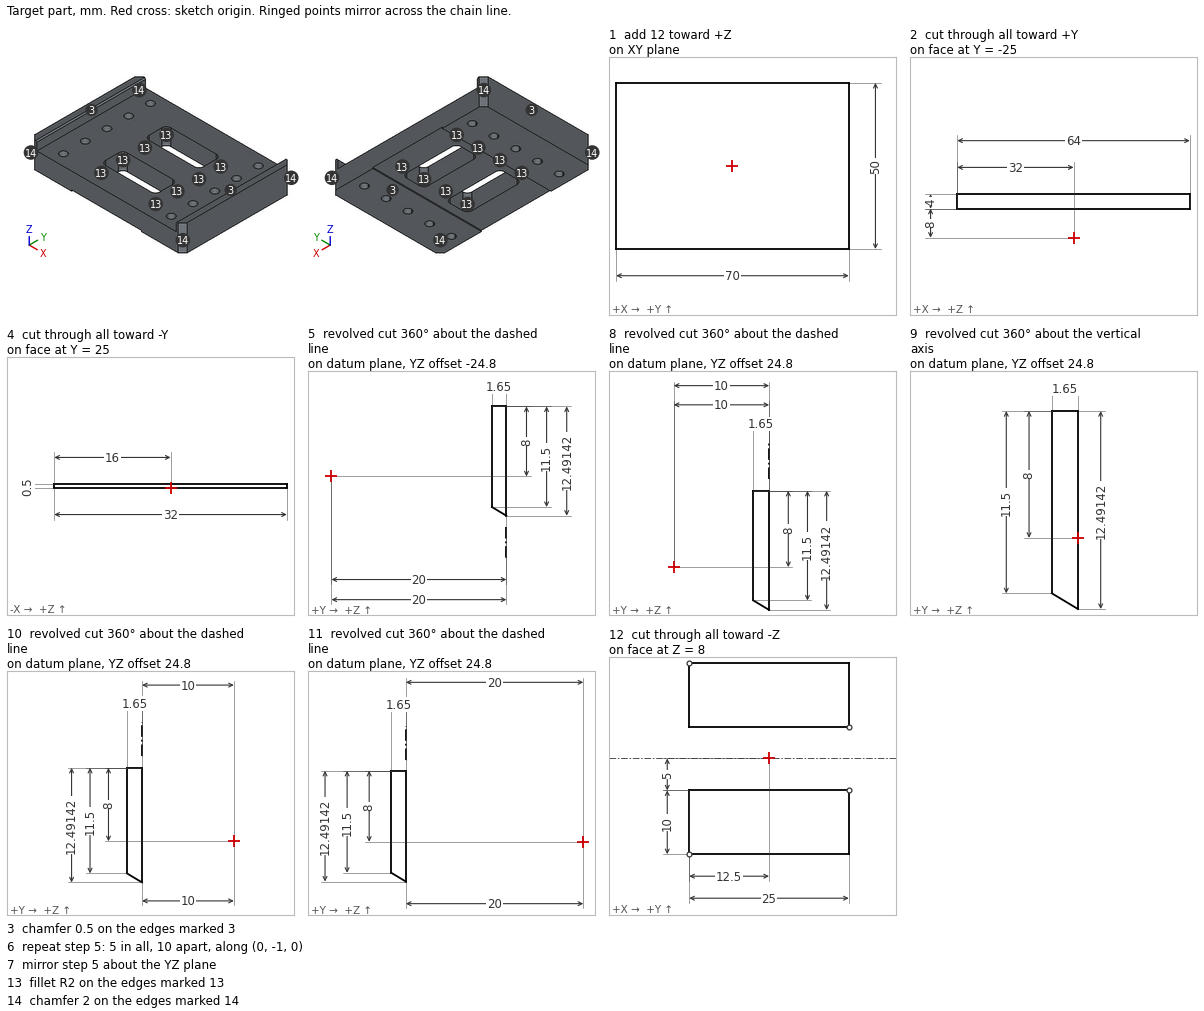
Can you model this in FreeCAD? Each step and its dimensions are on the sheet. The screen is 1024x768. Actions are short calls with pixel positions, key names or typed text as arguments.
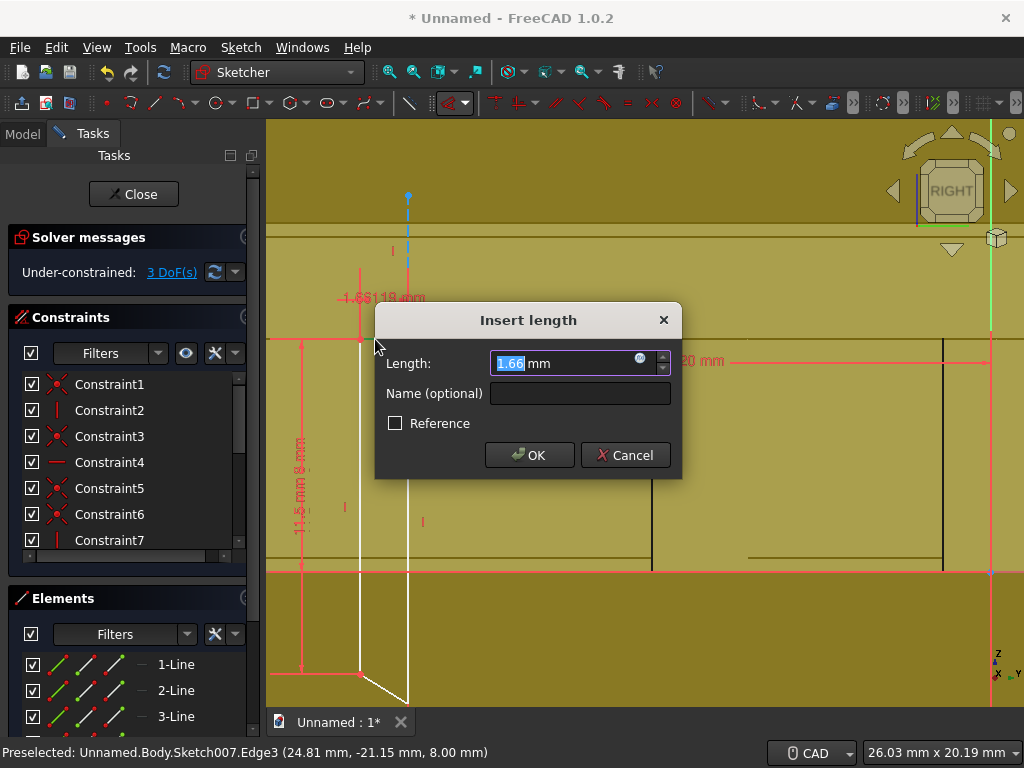
text(1.65)
key(Return)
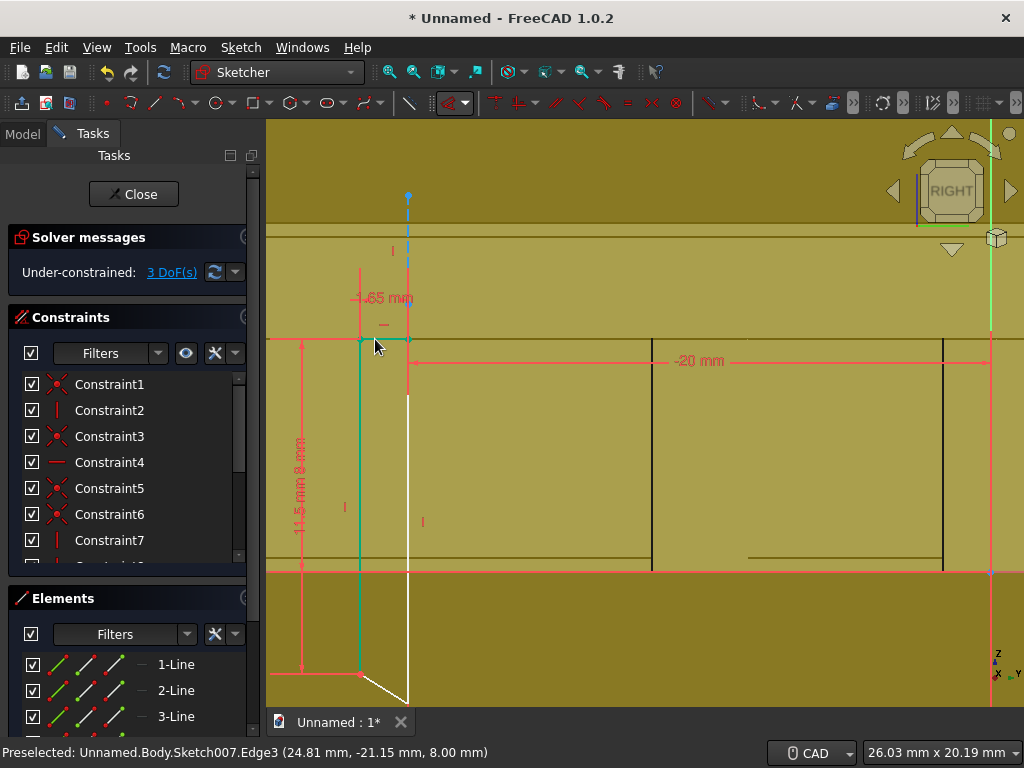
click(408, 449)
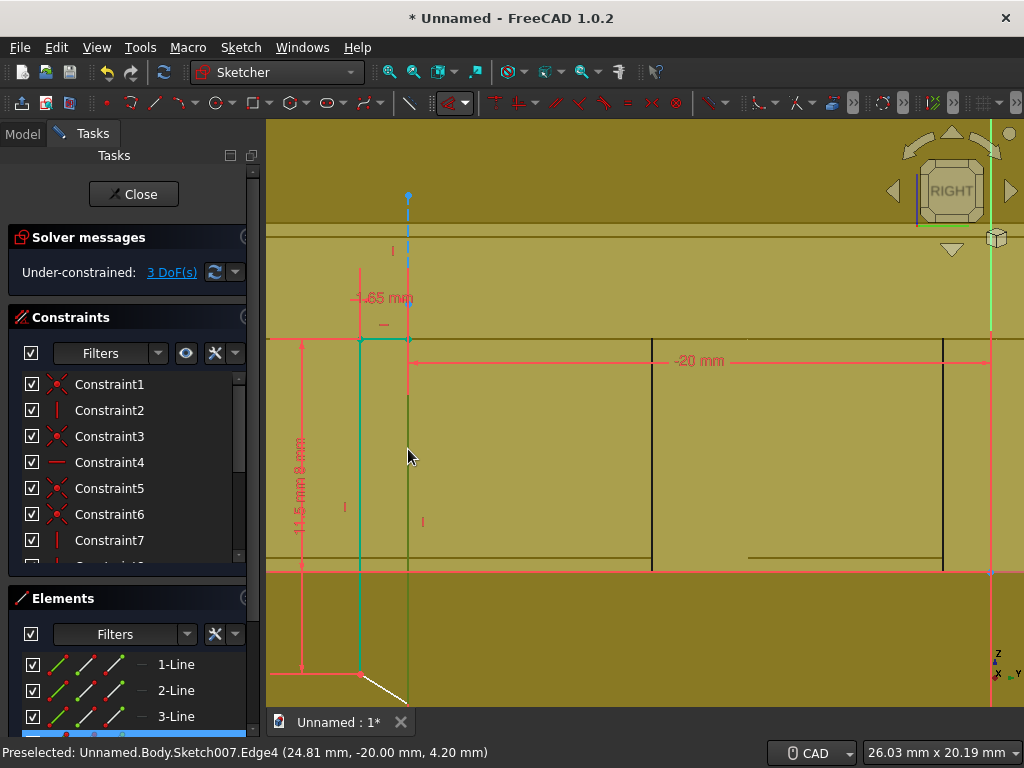
click(468, 104)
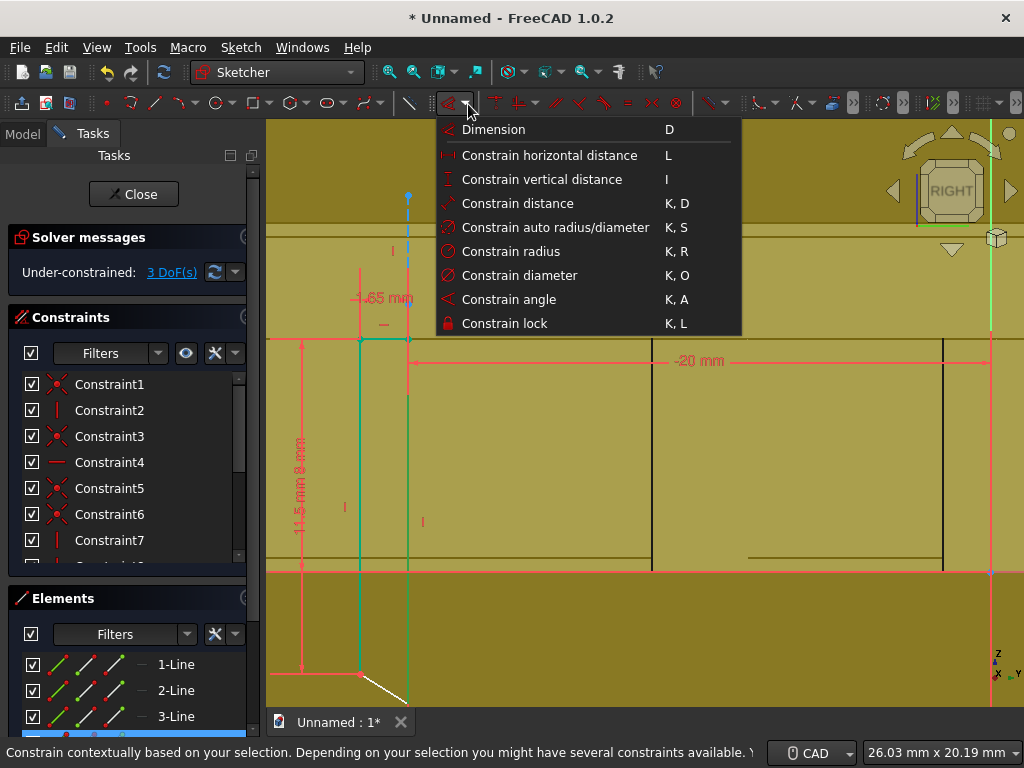
click(589, 179)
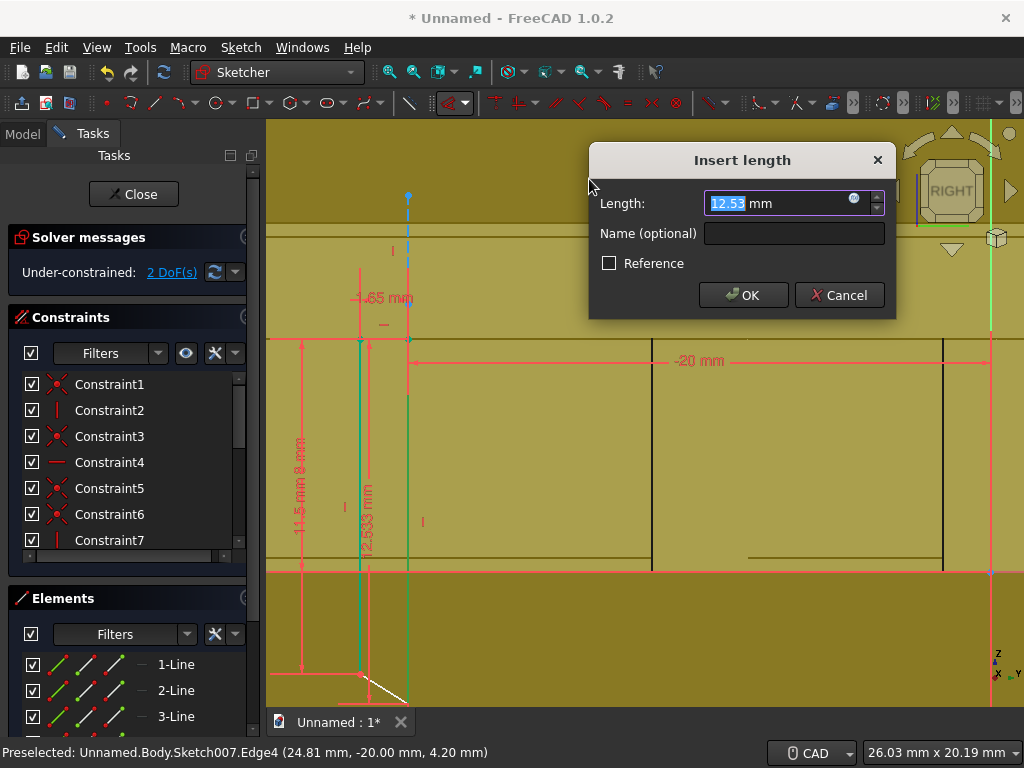
text(12.49142)
key(Return)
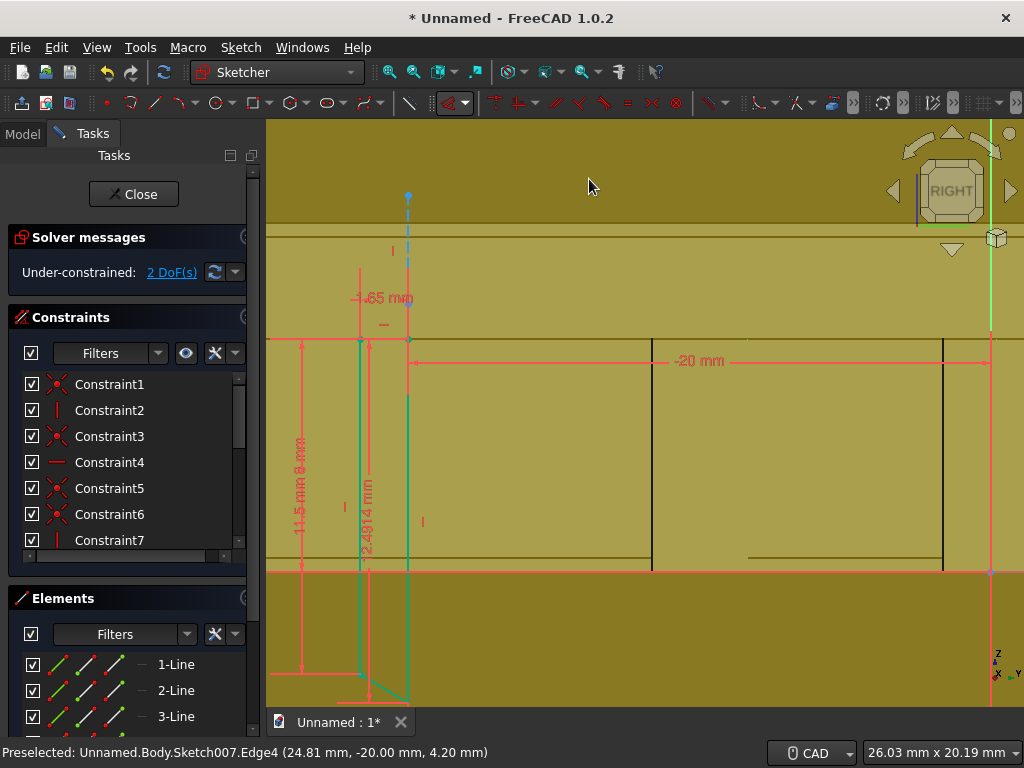
click(134, 194)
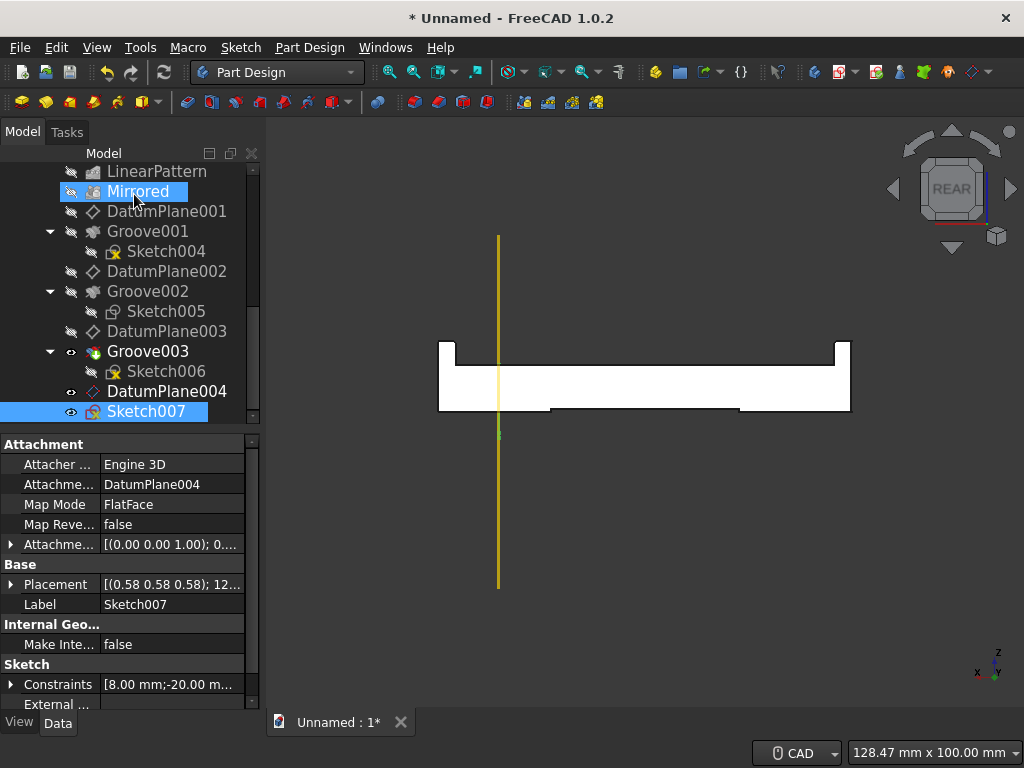
click(236, 102)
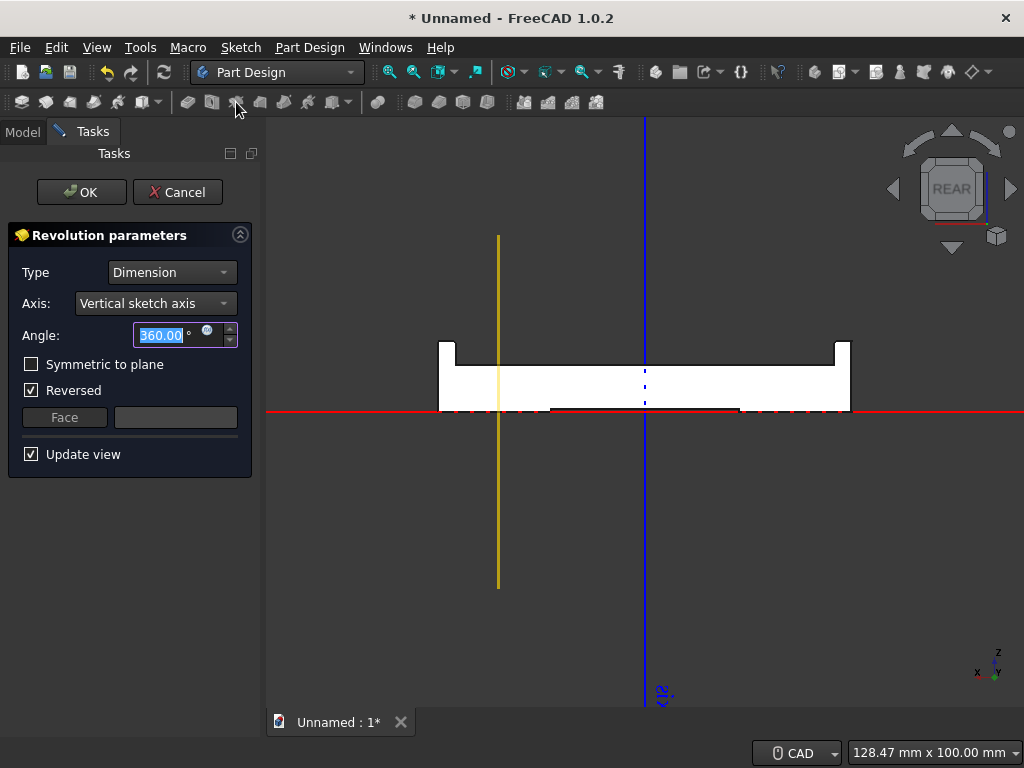
click(156, 304)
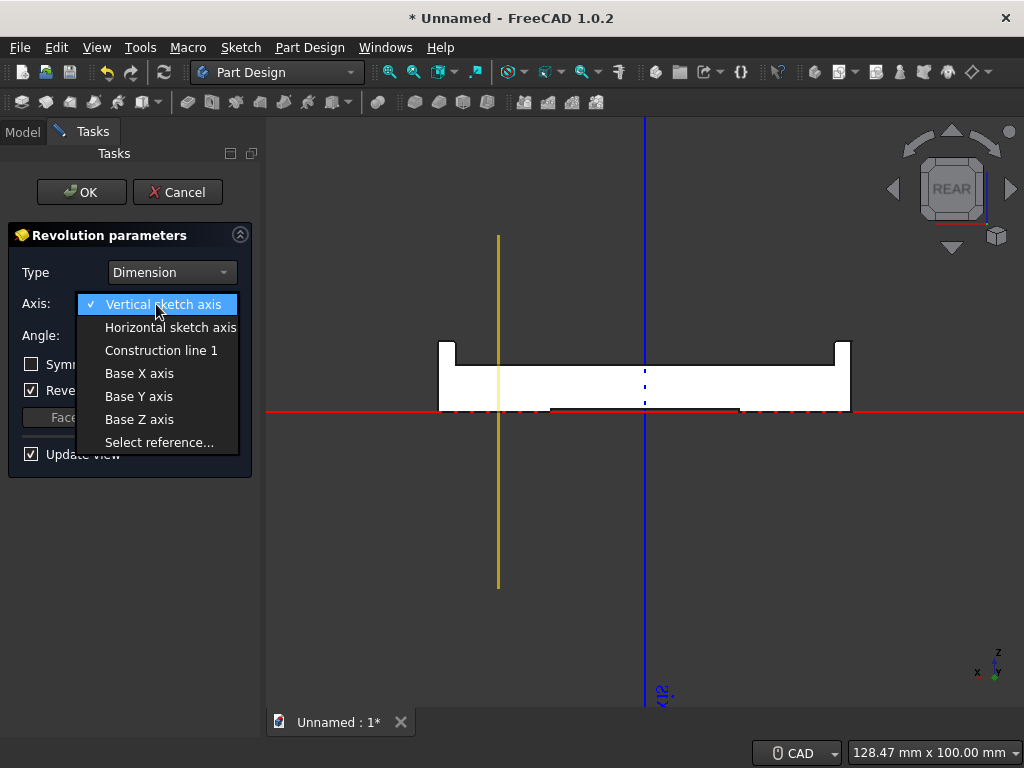
click(156, 350)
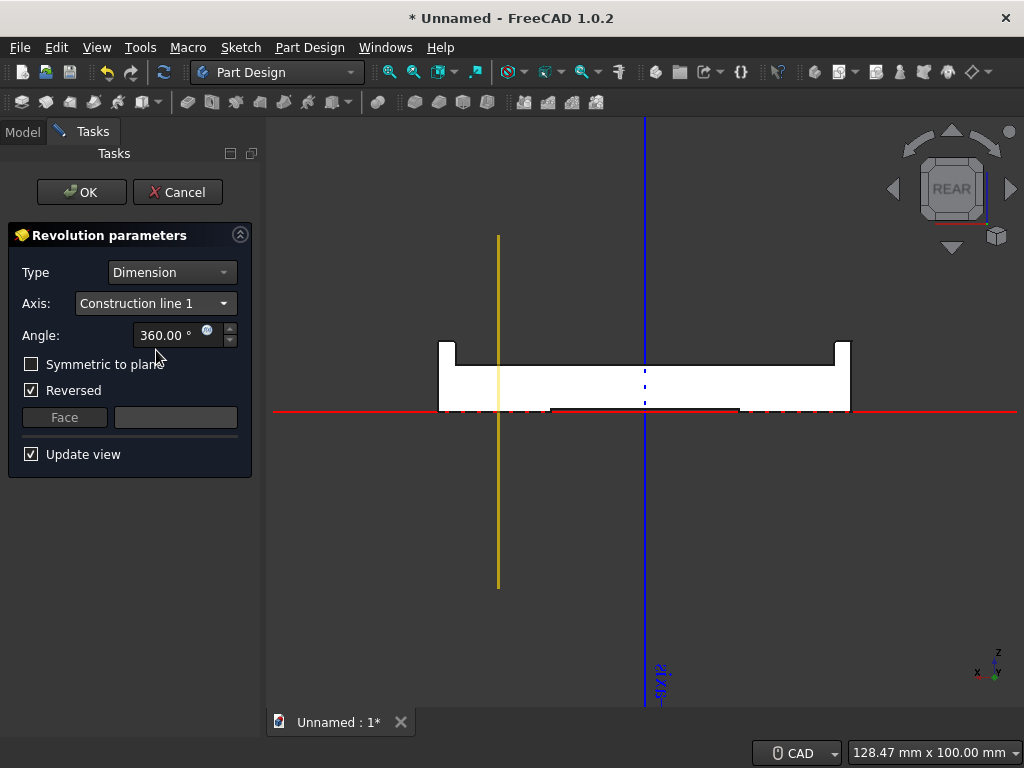
click(82, 192)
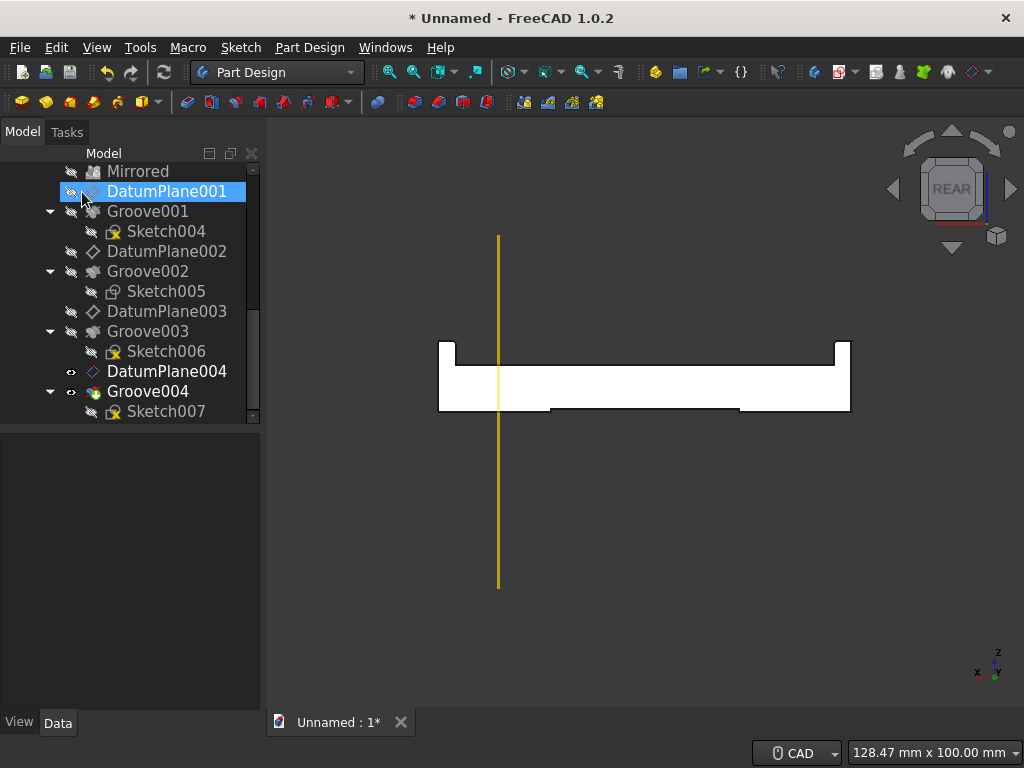
click(116, 372)
key(space)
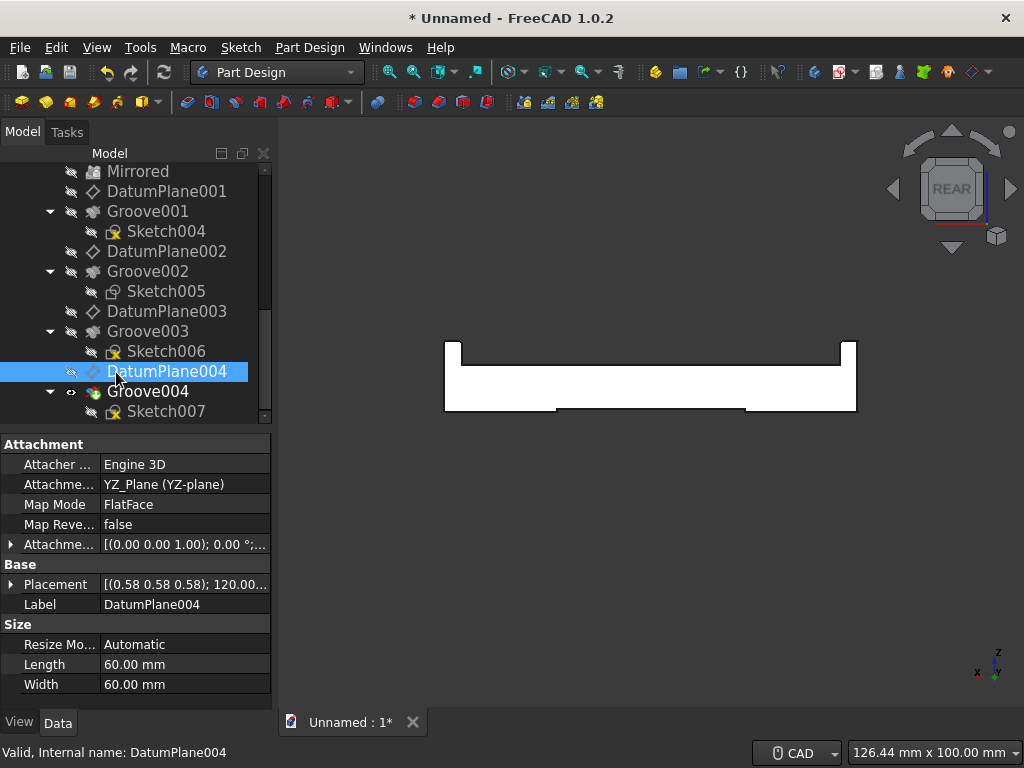
key(0)